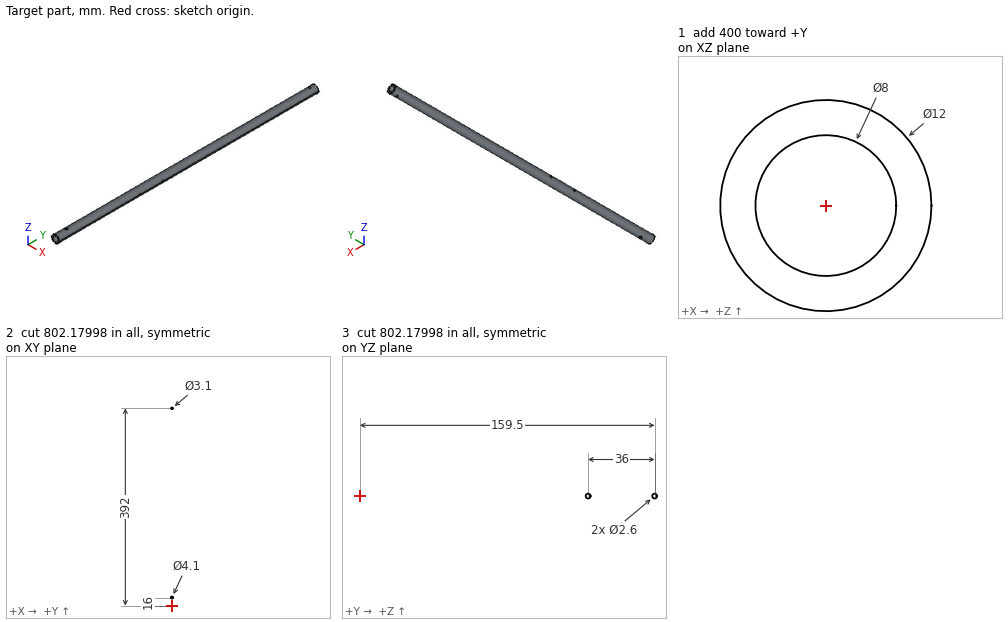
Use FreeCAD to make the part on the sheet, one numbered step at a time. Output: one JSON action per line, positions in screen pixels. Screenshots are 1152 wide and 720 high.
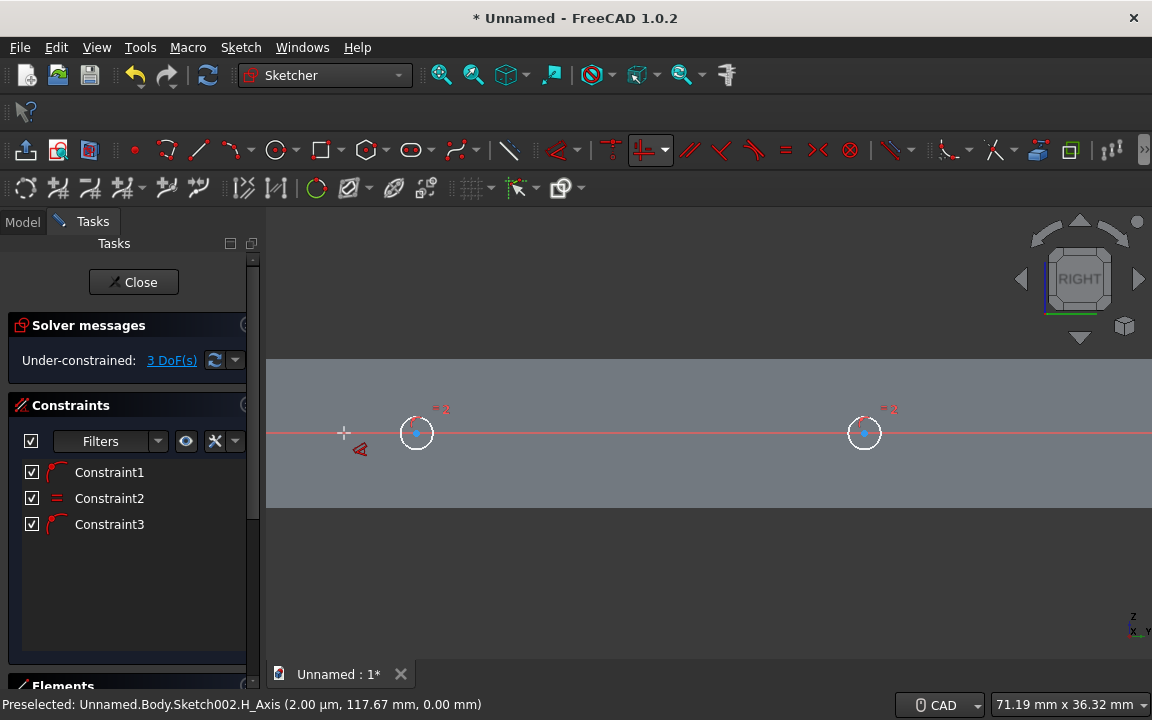
{"action": "scroll", "coordinate": [876, 422], "scroll_direction": "up", "scroll_amount": 2}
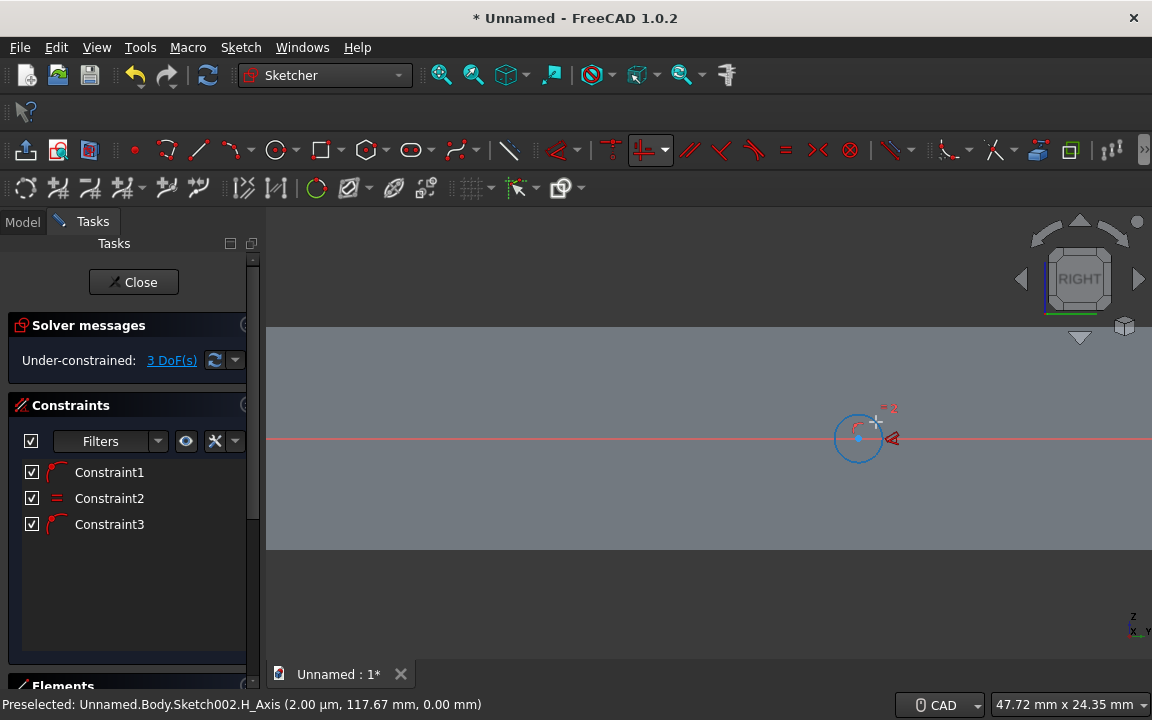
{"action": "left_click", "coordinate": [876, 422]}
{"action": "left_click", "coordinate": [899, 400]}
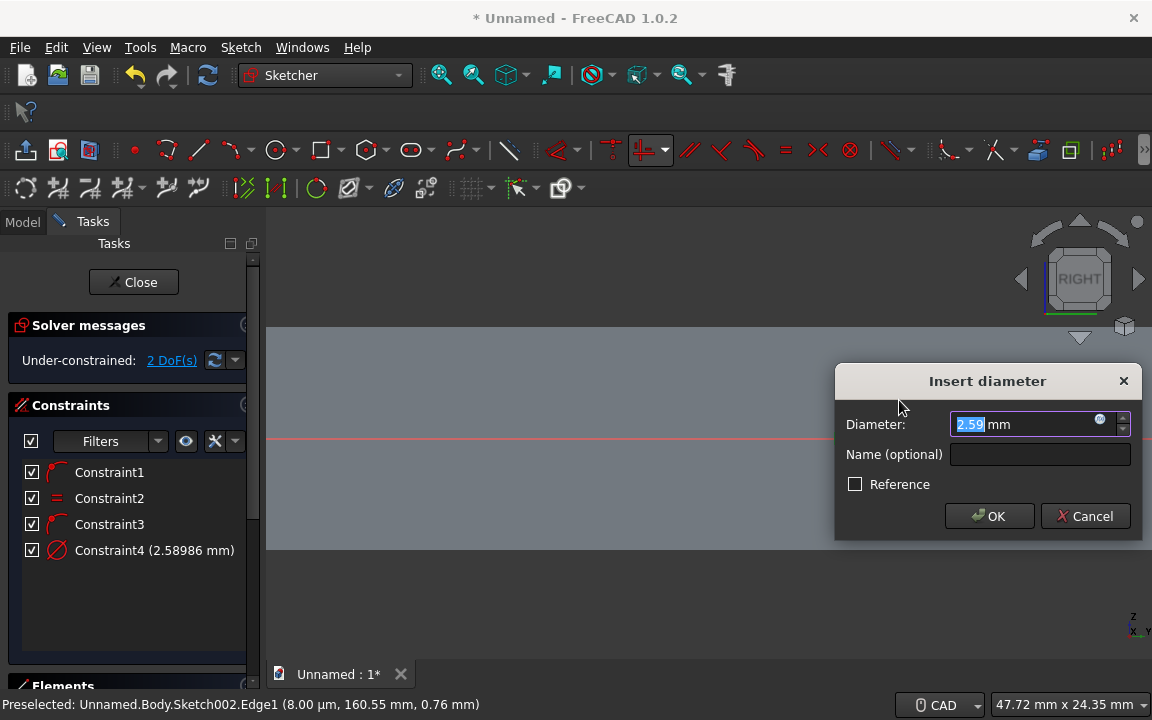
{"action": "type", "text": "2.6"}
{"action": "key", "text": "Return"}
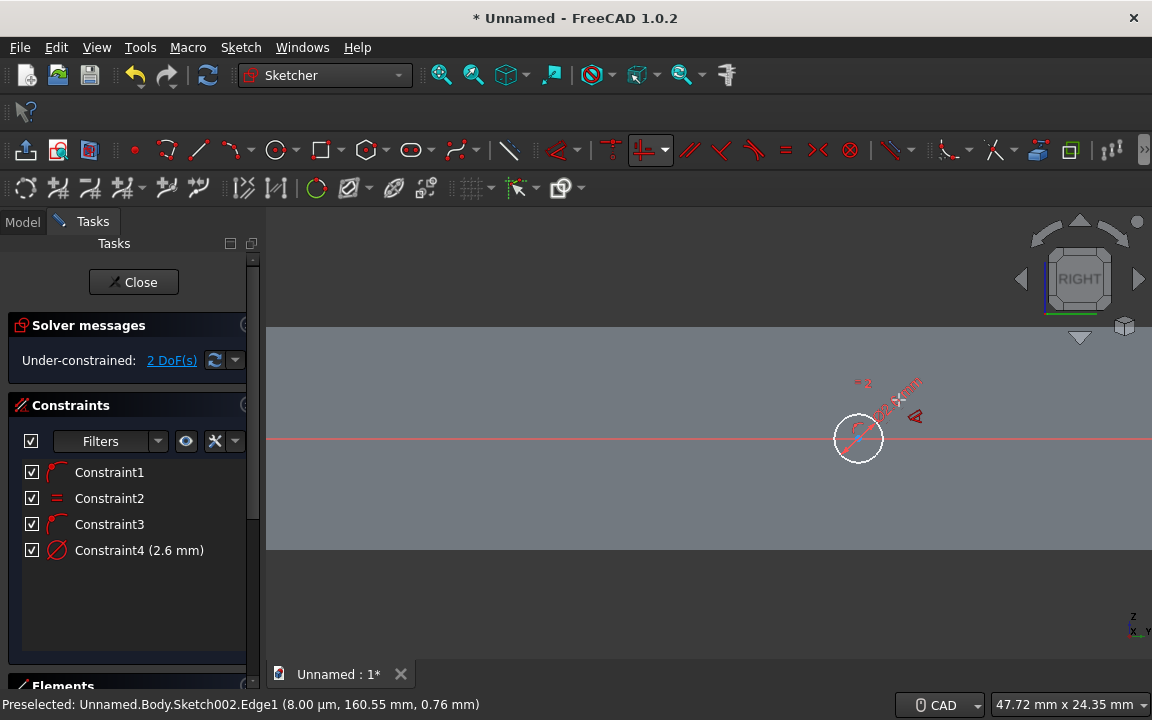
{"action": "left_click", "coordinate": [859, 439]}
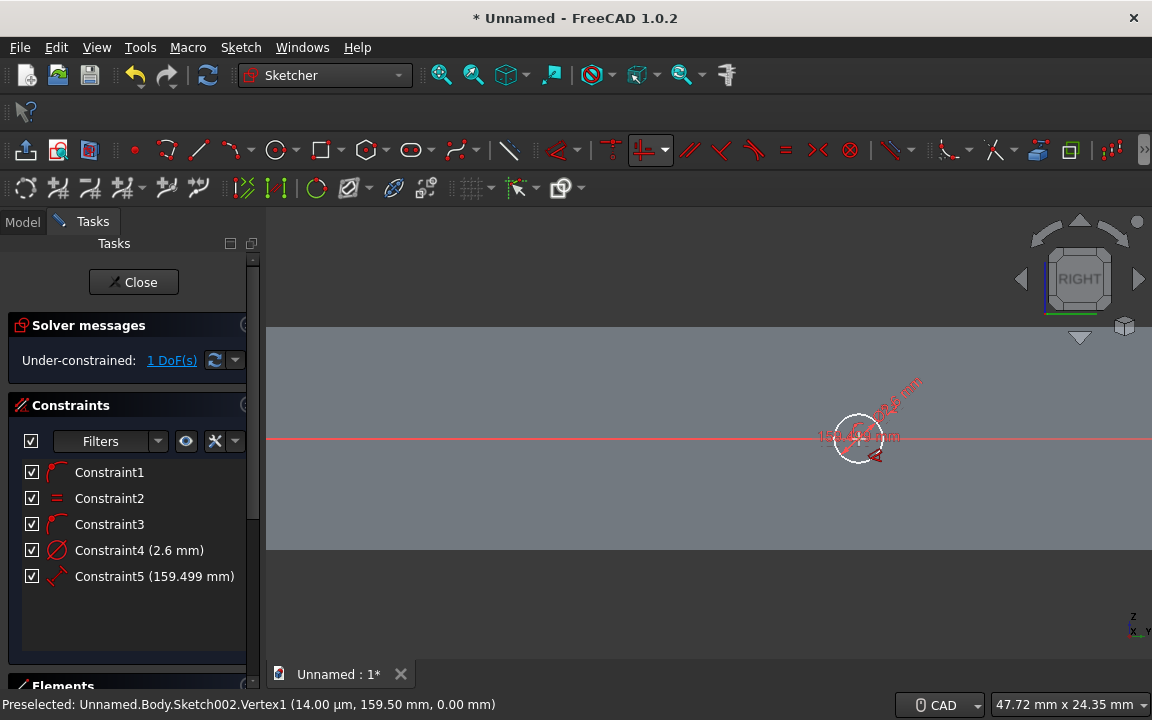
{"action": "scroll", "coordinate": [877, 422], "scroll_direction": "down", "scroll_amount": 2}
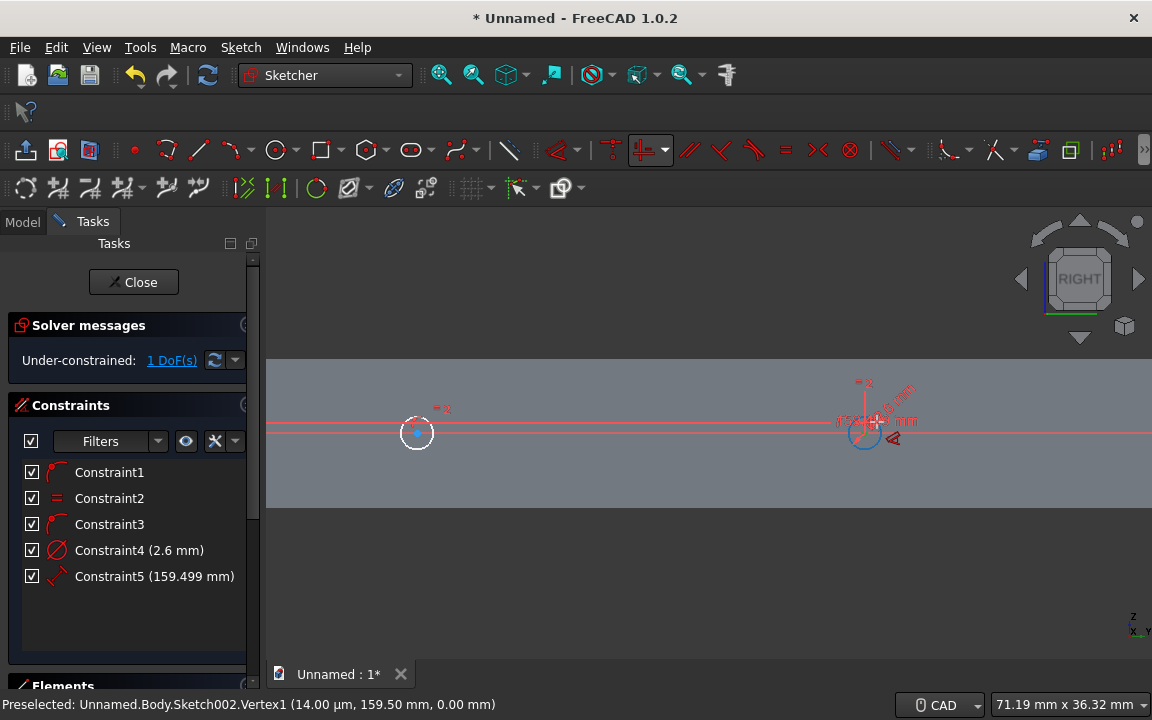
{"action": "left_click", "coordinate": [417, 433]}
{"action": "left_click", "coordinate": [641, 467]}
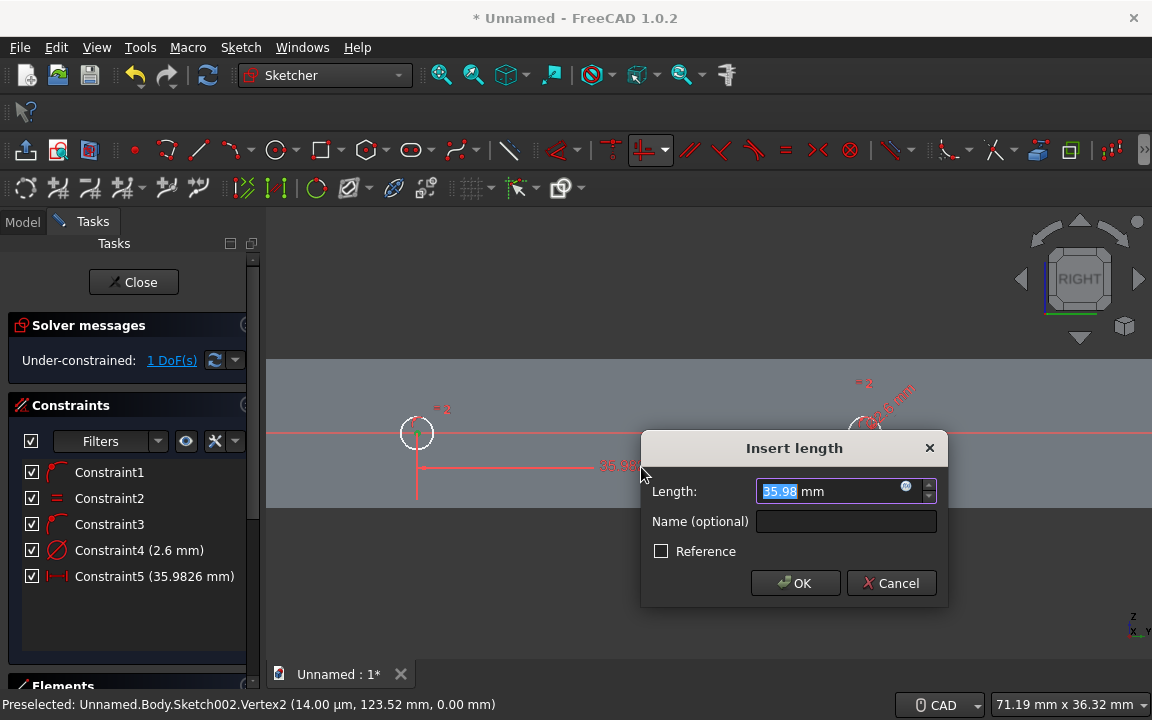
{"action": "type", "text": "36"}
{"action": "key", "text": "Return"}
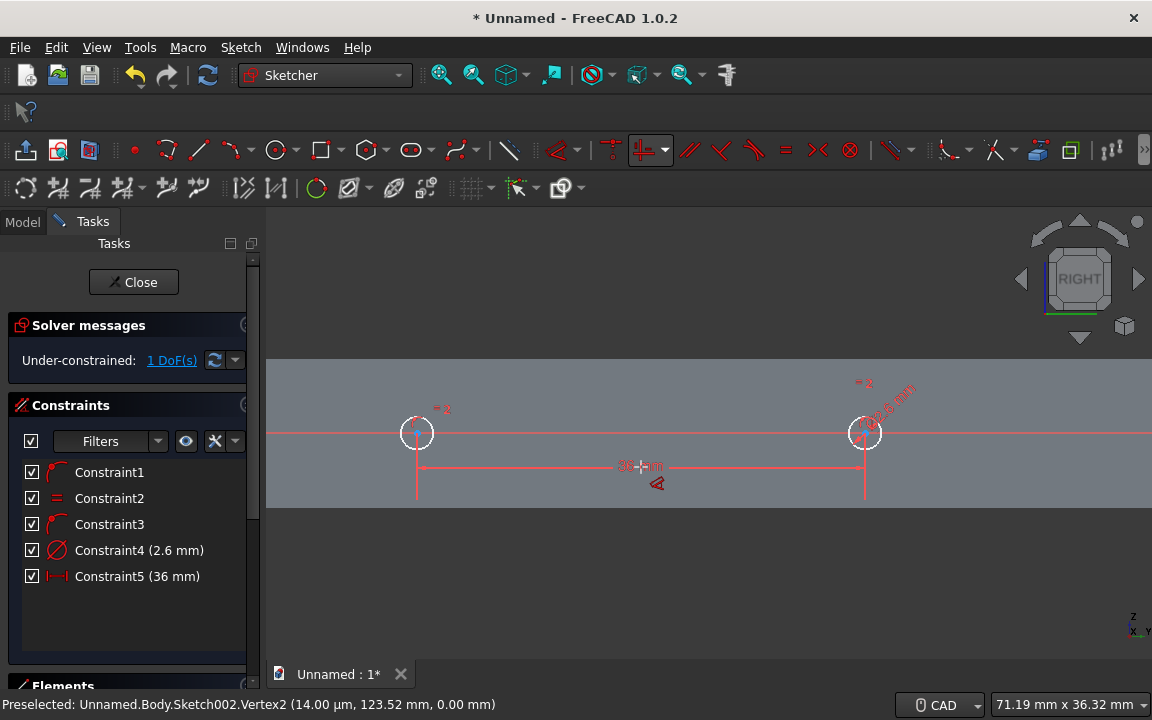
{"action": "left_click", "coordinate": [865, 433]}
{"action": "left_click", "coordinate": [448, 467]}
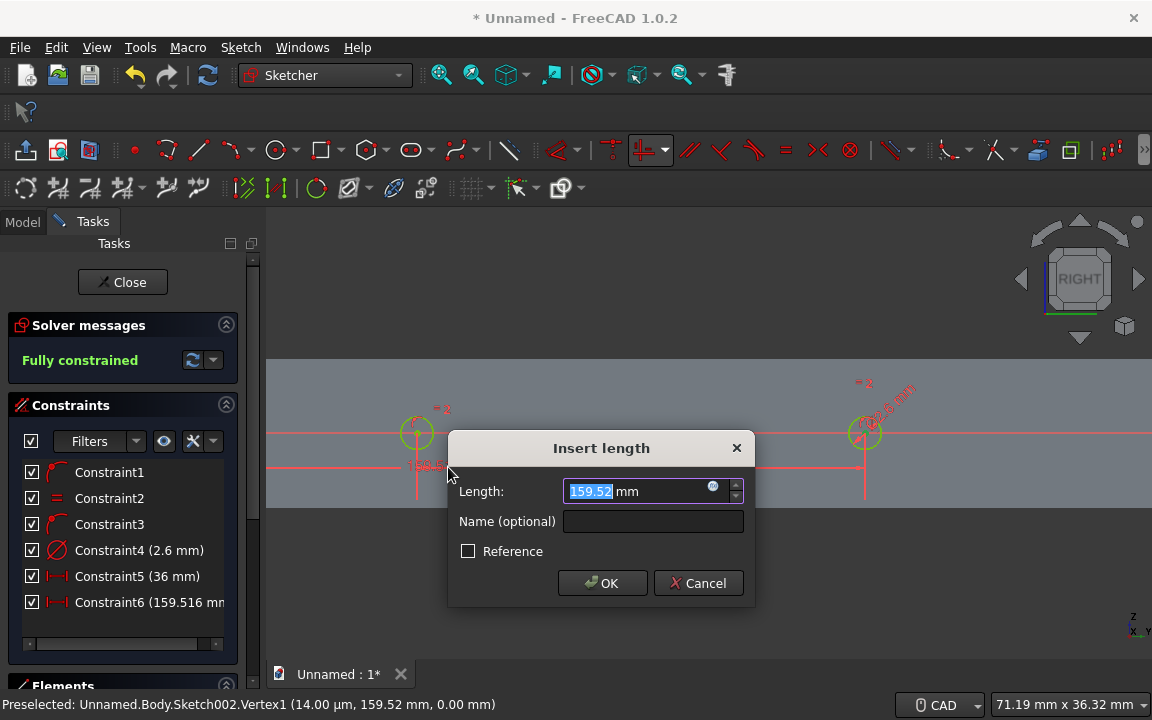
{"action": "type", "text": "159.5"}
{"action": "key", "text": "Return"}
{"action": "key", "text": "Escape"}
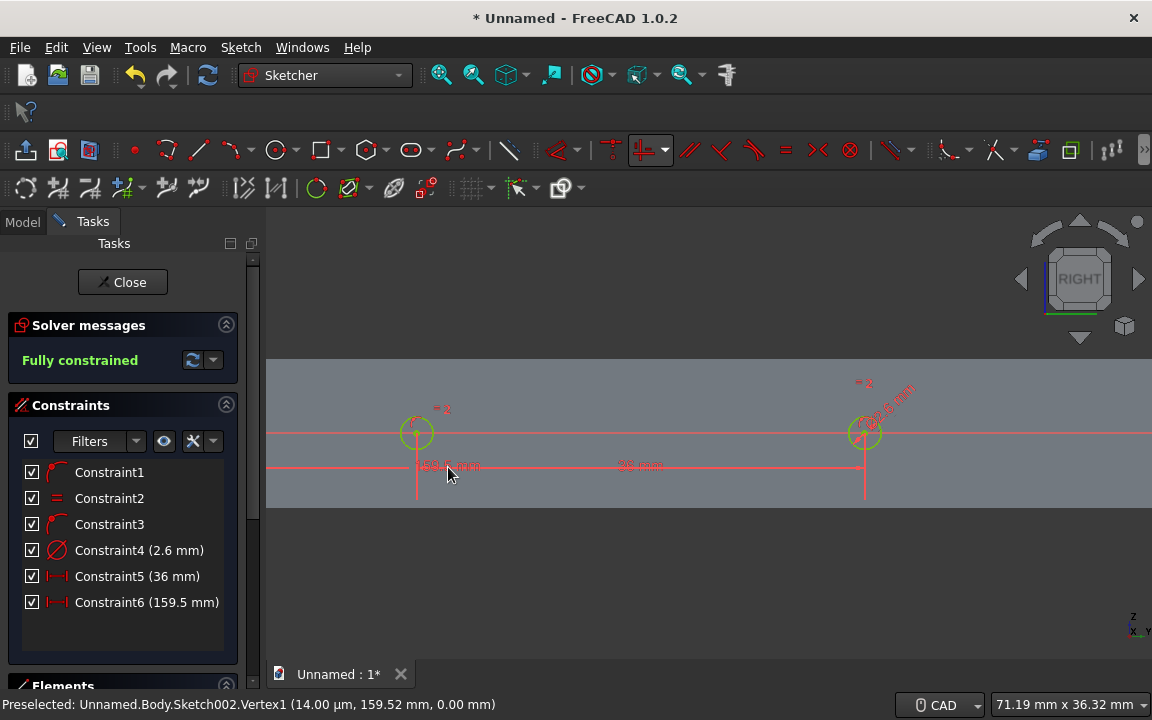
{"action": "left_click", "coordinate": [123, 282]}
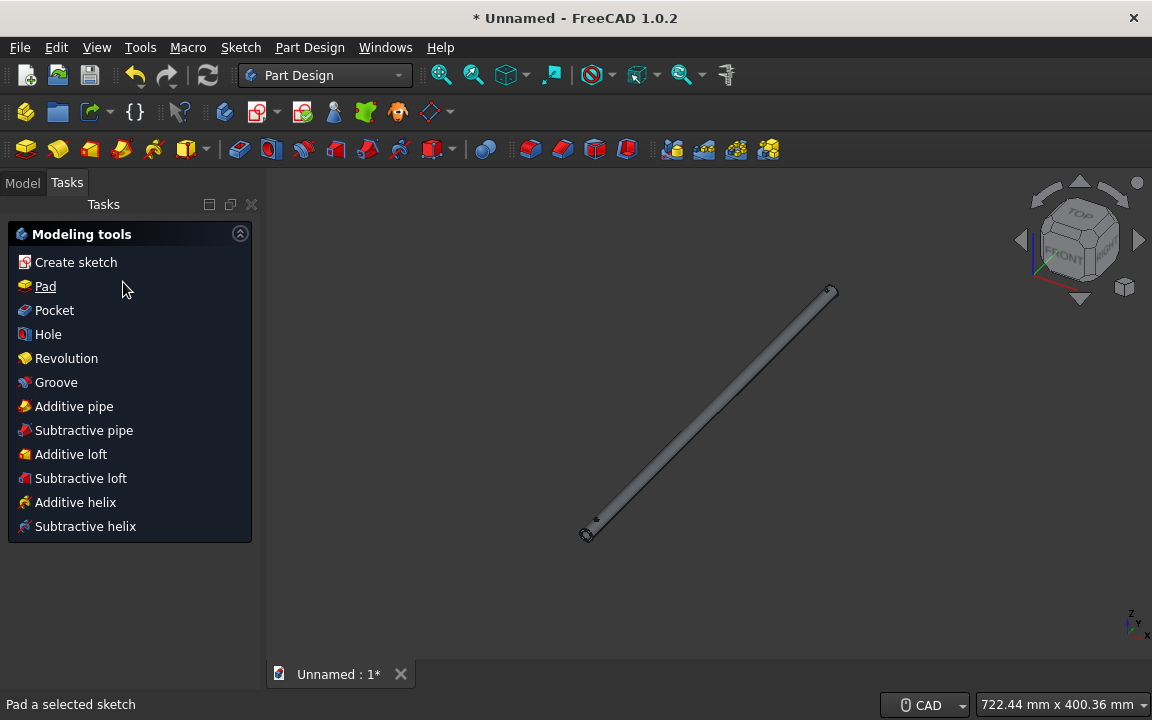
{"action": "left_click", "coordinate": [240, 150]}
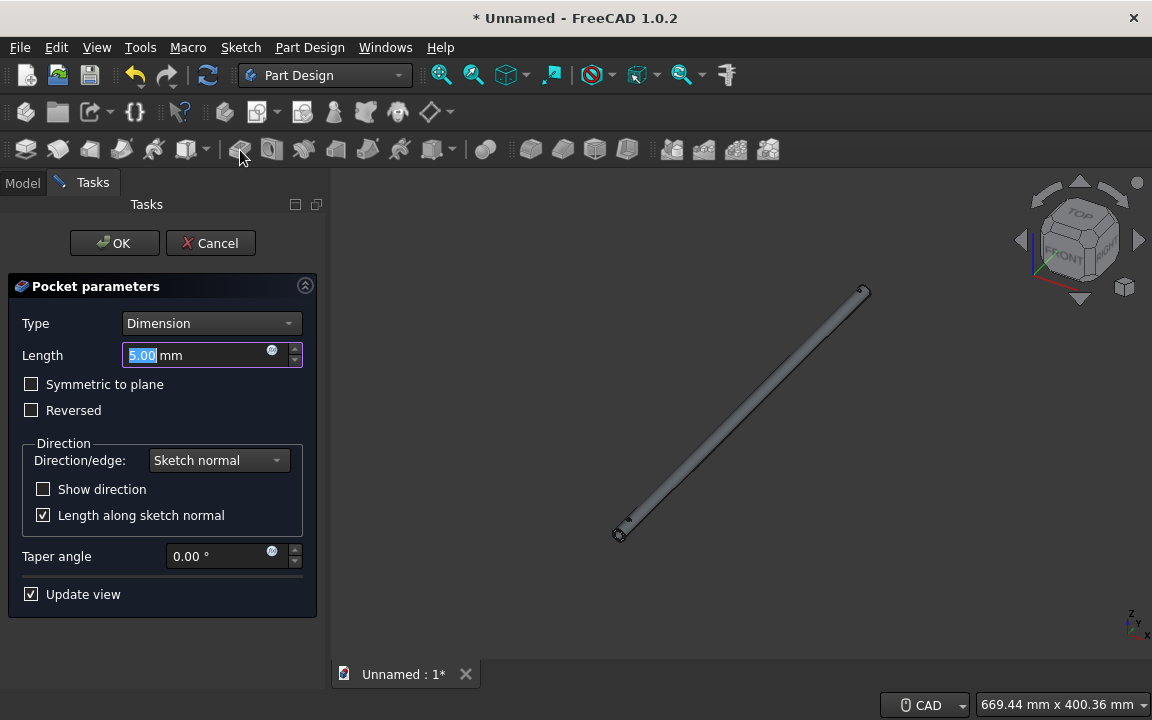
{"action": "type", "text": "802.17998"}
{"action": "key", "text": "Tab"}